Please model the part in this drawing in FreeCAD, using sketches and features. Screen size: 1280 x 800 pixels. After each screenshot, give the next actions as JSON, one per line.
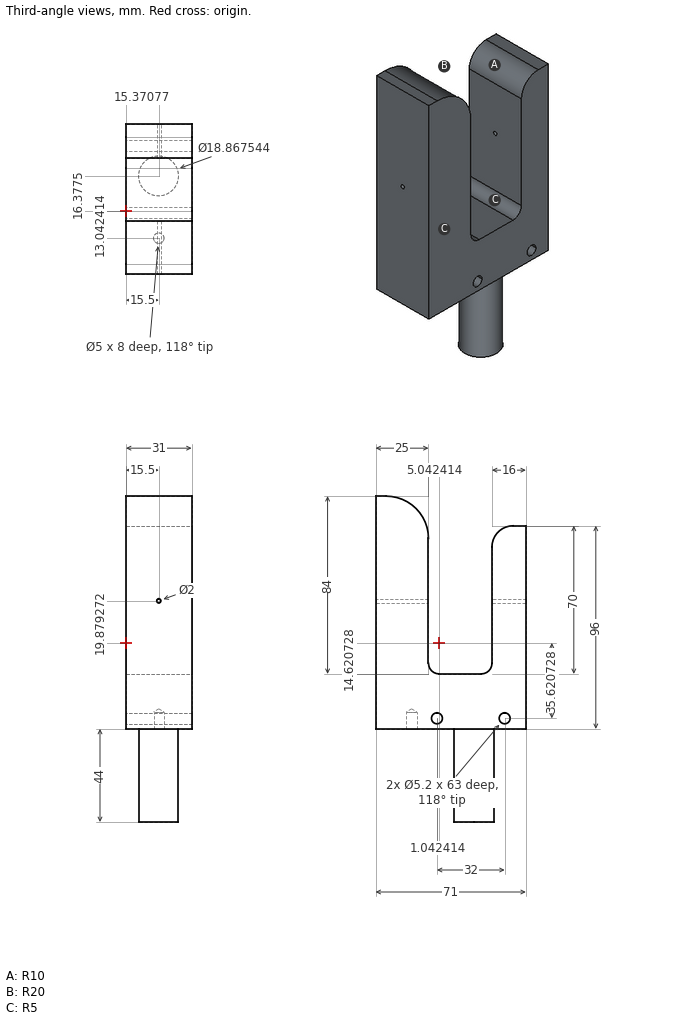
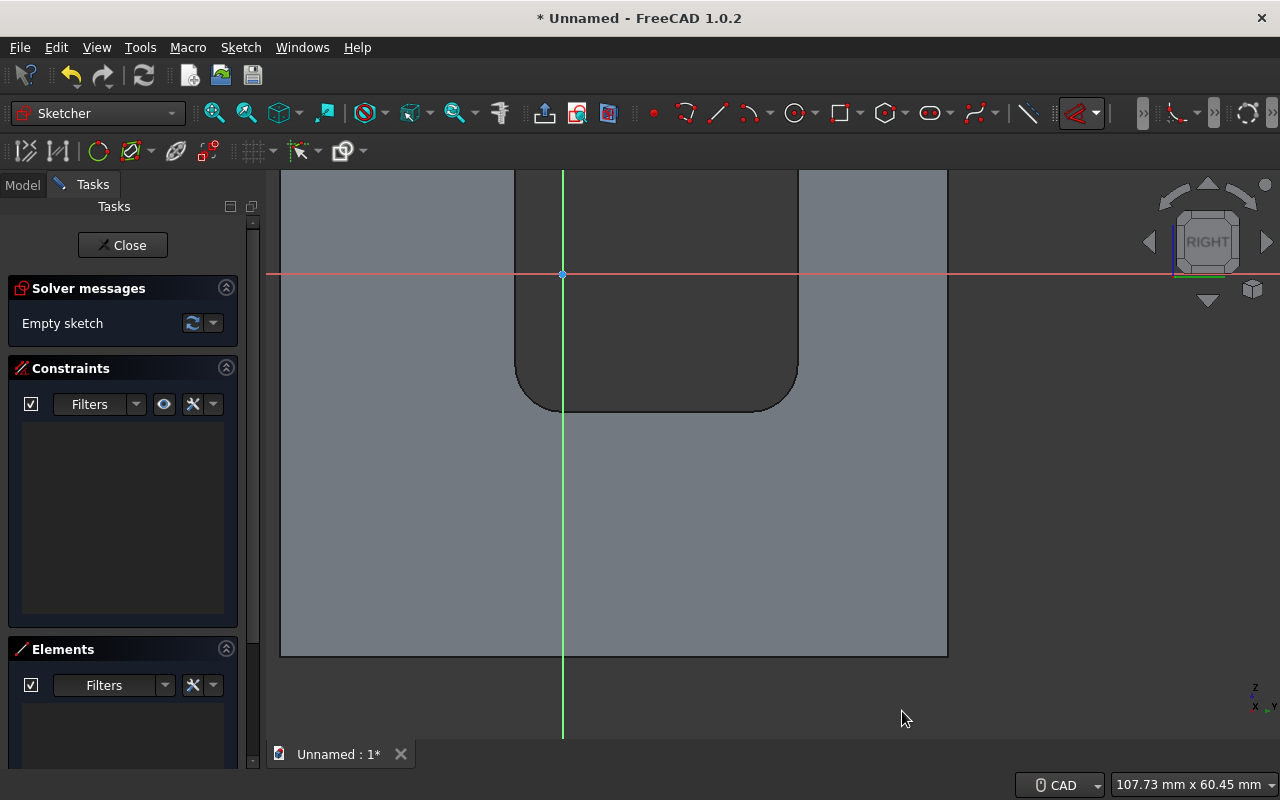
{"action": "left_click", "coordinate": [796, 114]}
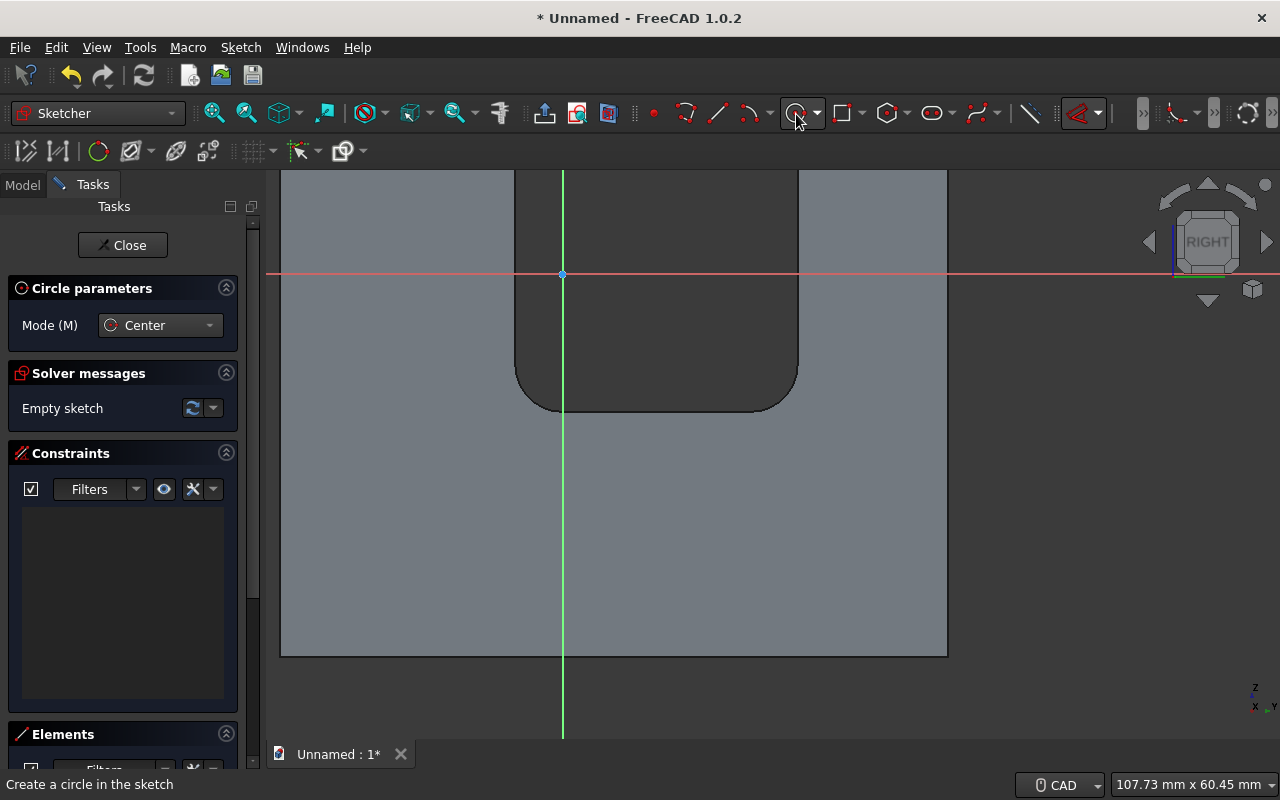
{"action": "left_click", "coordinate": [854, 610]}
{"action": "mouse_move", "coordinate": [871, 592]}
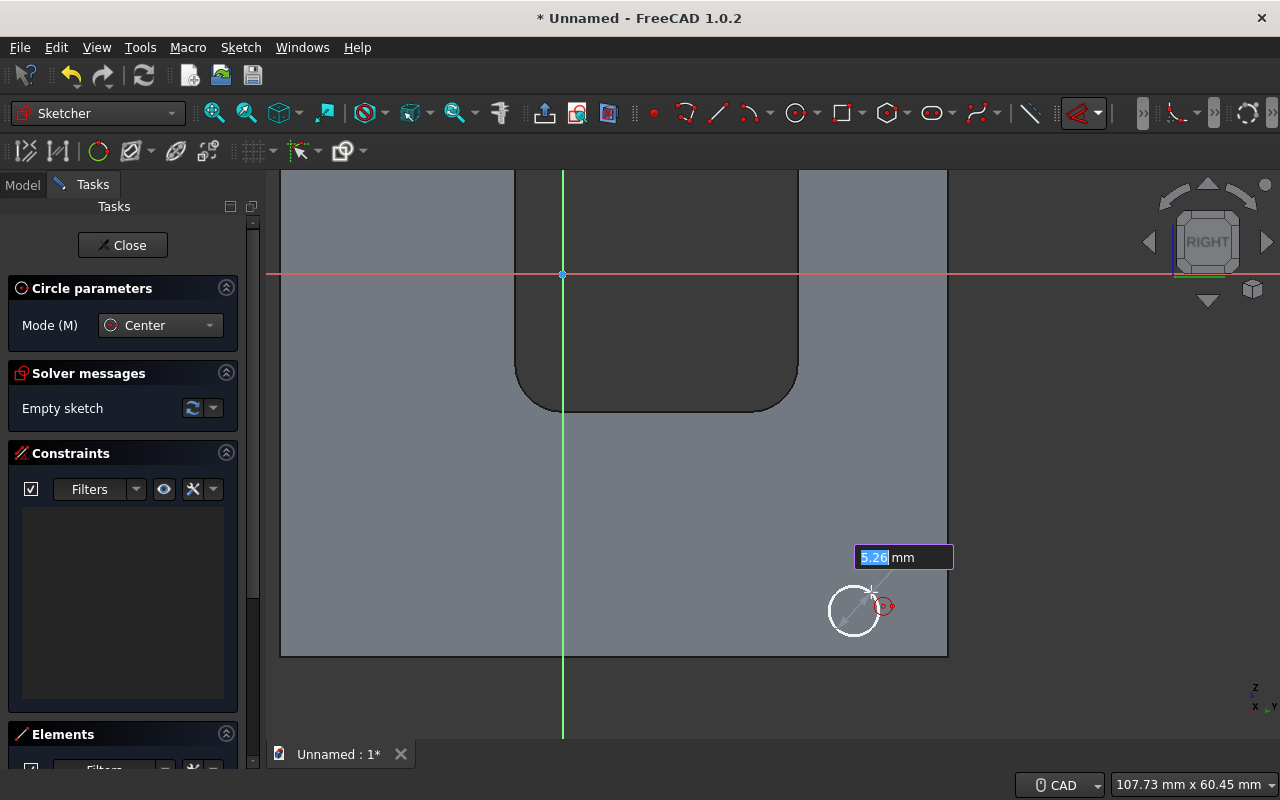
{"action": "type", "text": "5.2"}
{"action": "key", "text": "Return"}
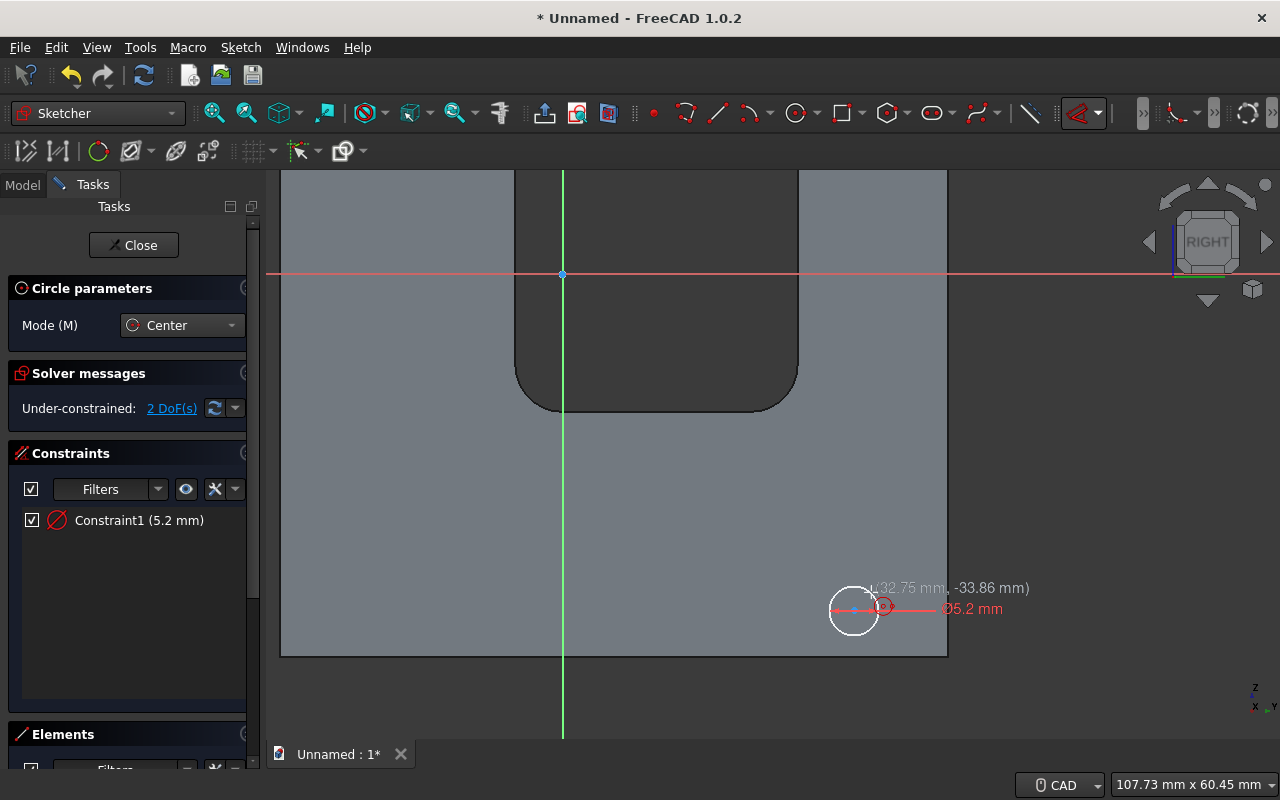
{"action": "scroll", "coordinate": [553, 610], "scroll_direction": "up", "scroll_amount": 3}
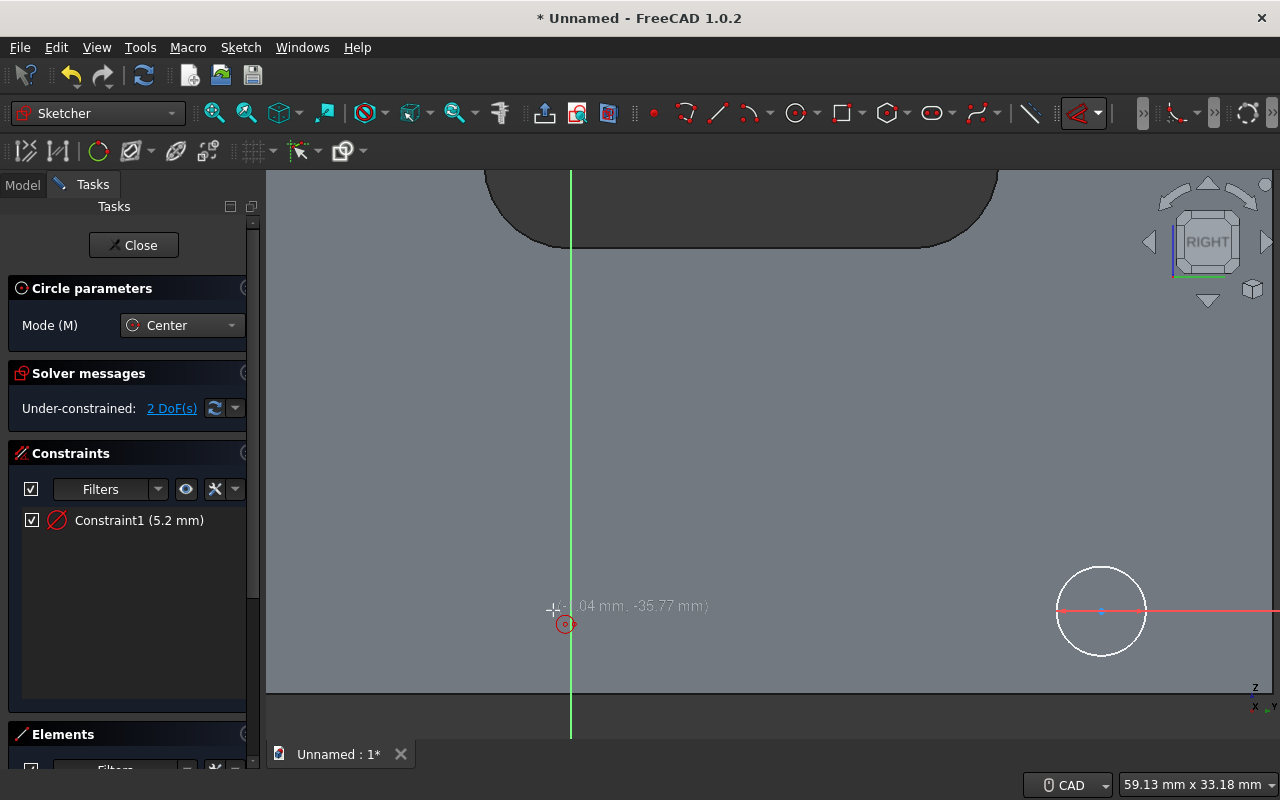
{"action": "left_click", "coordinate": [553, 609]}
{"action": "mouse_move", "coordinate": [521, 577]}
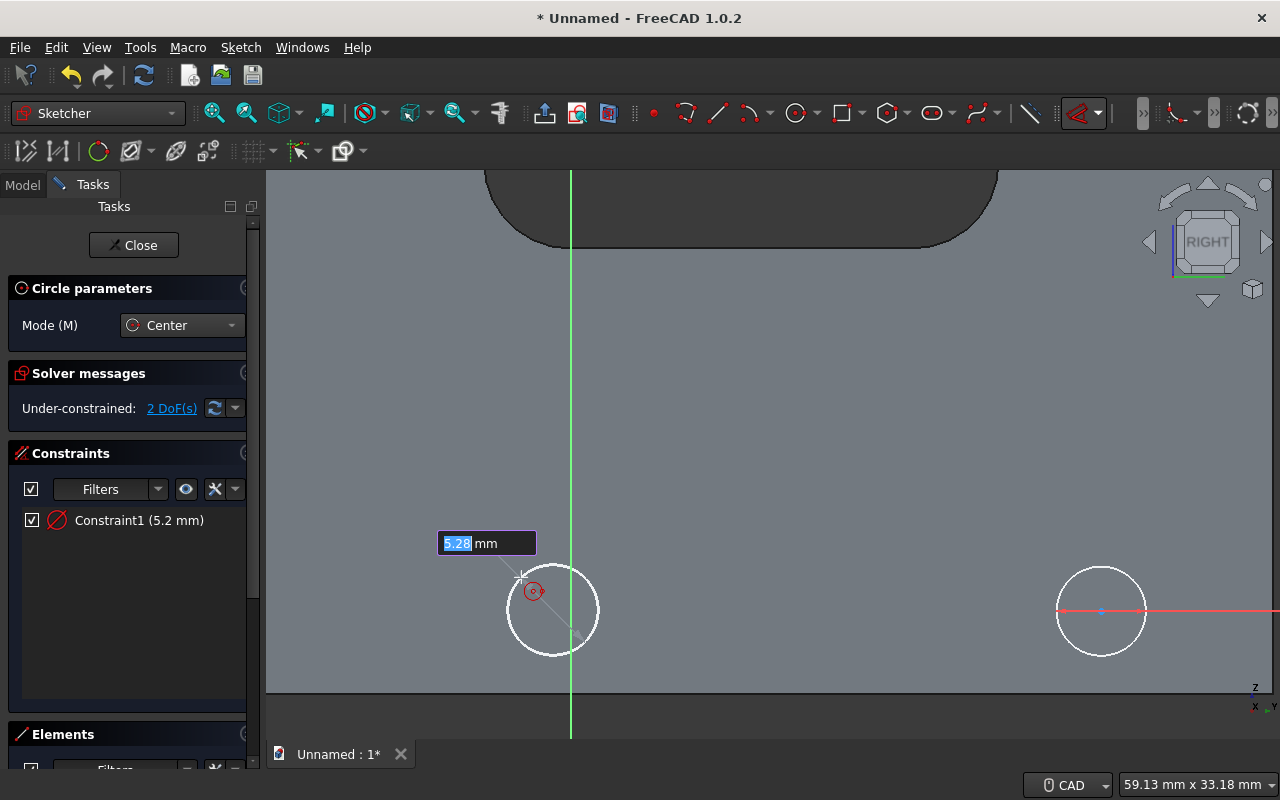
{"action": "type", "text": "5.2"}
{"action": "key", "text": "Return"}
{"action": "key", "text": "Escape"}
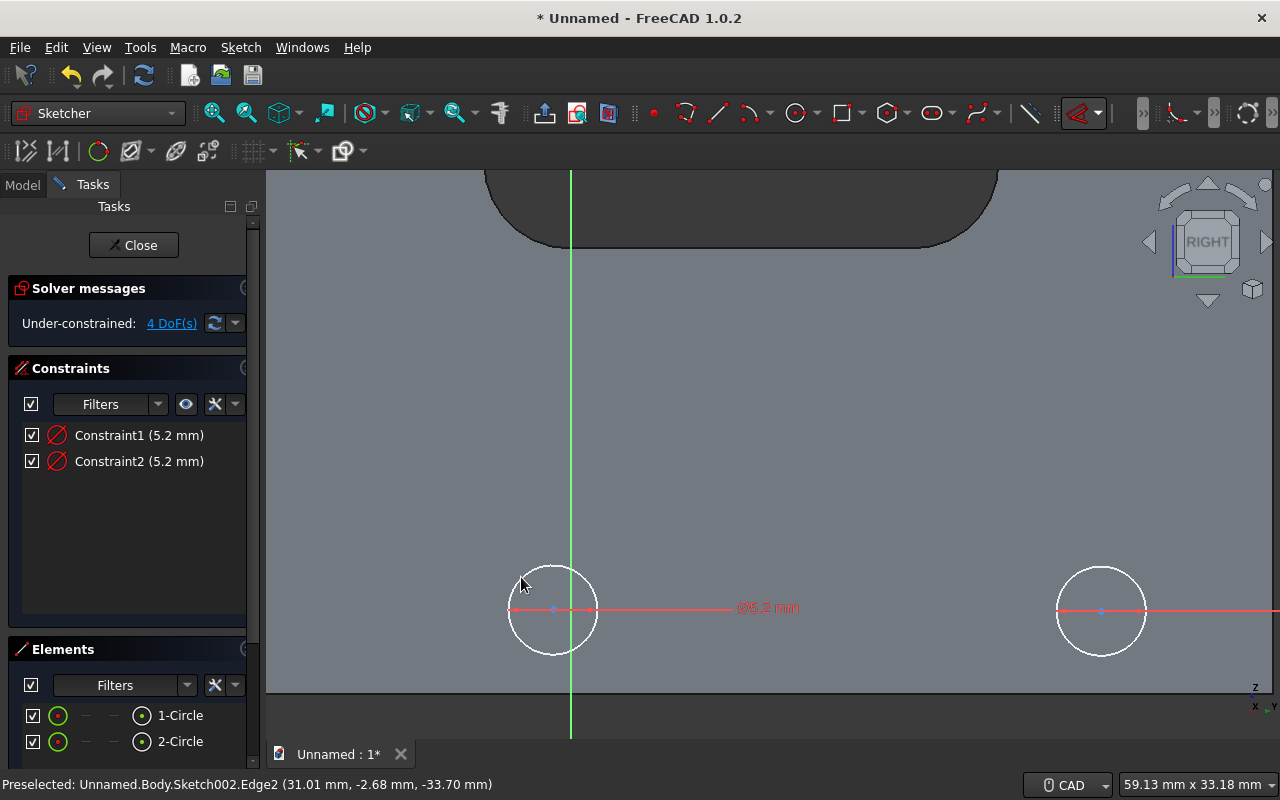
{"action": "left_click", "coordinate": [1101, 611]}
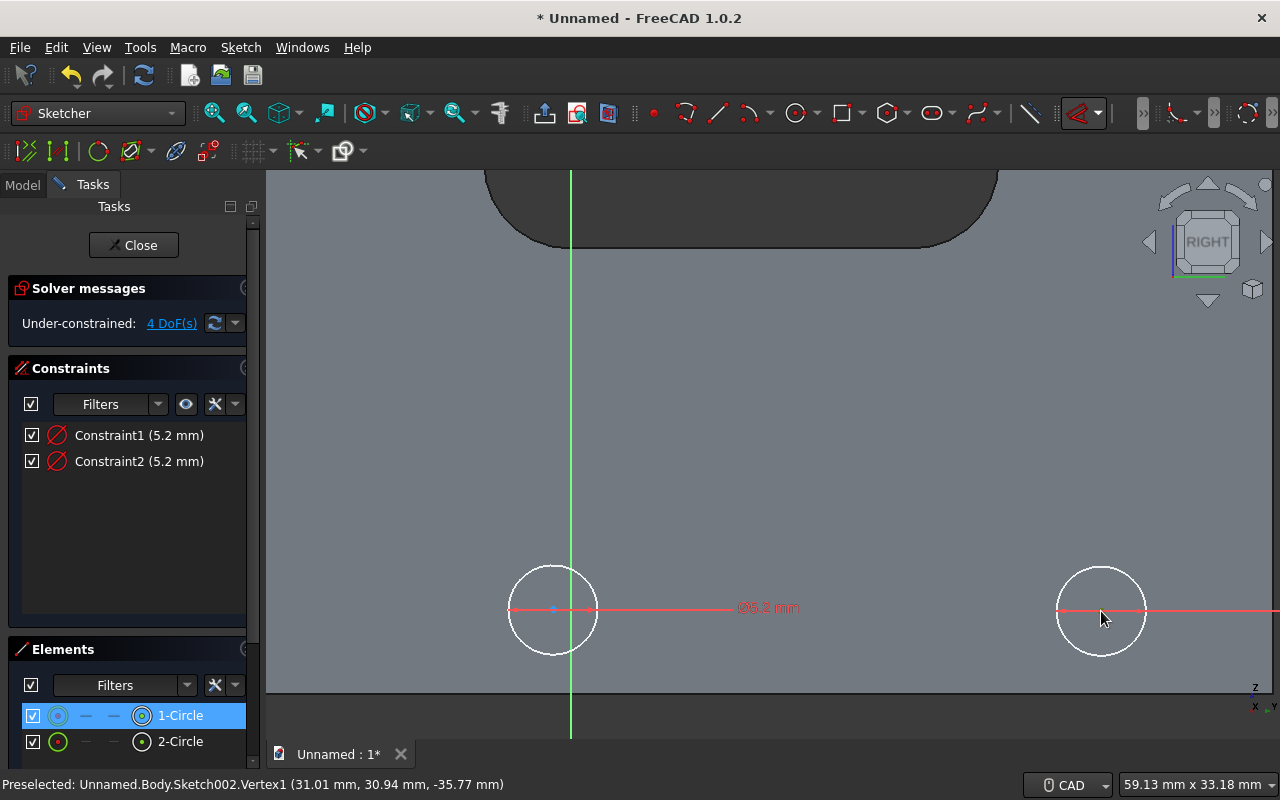
{"action": "left_click", "coordinate": [553, 610]}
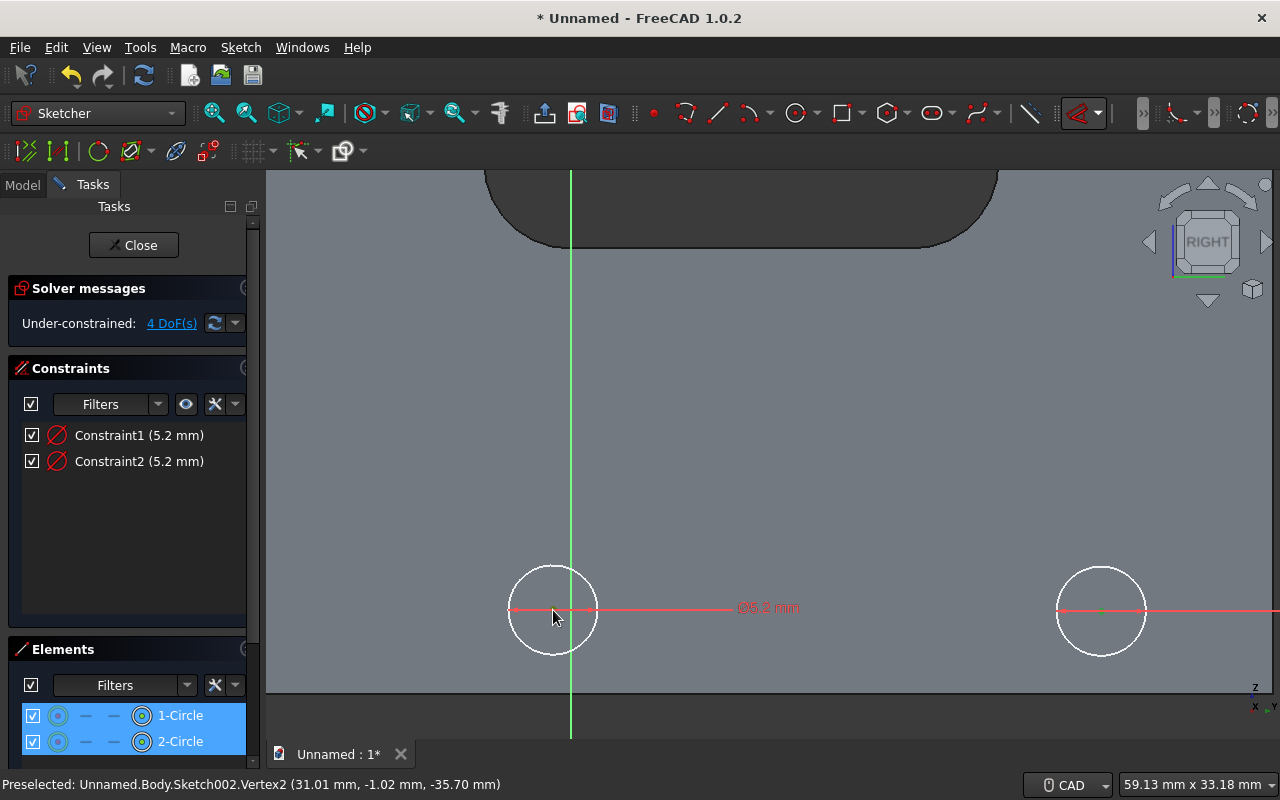
{"action": "key", "text": "h"}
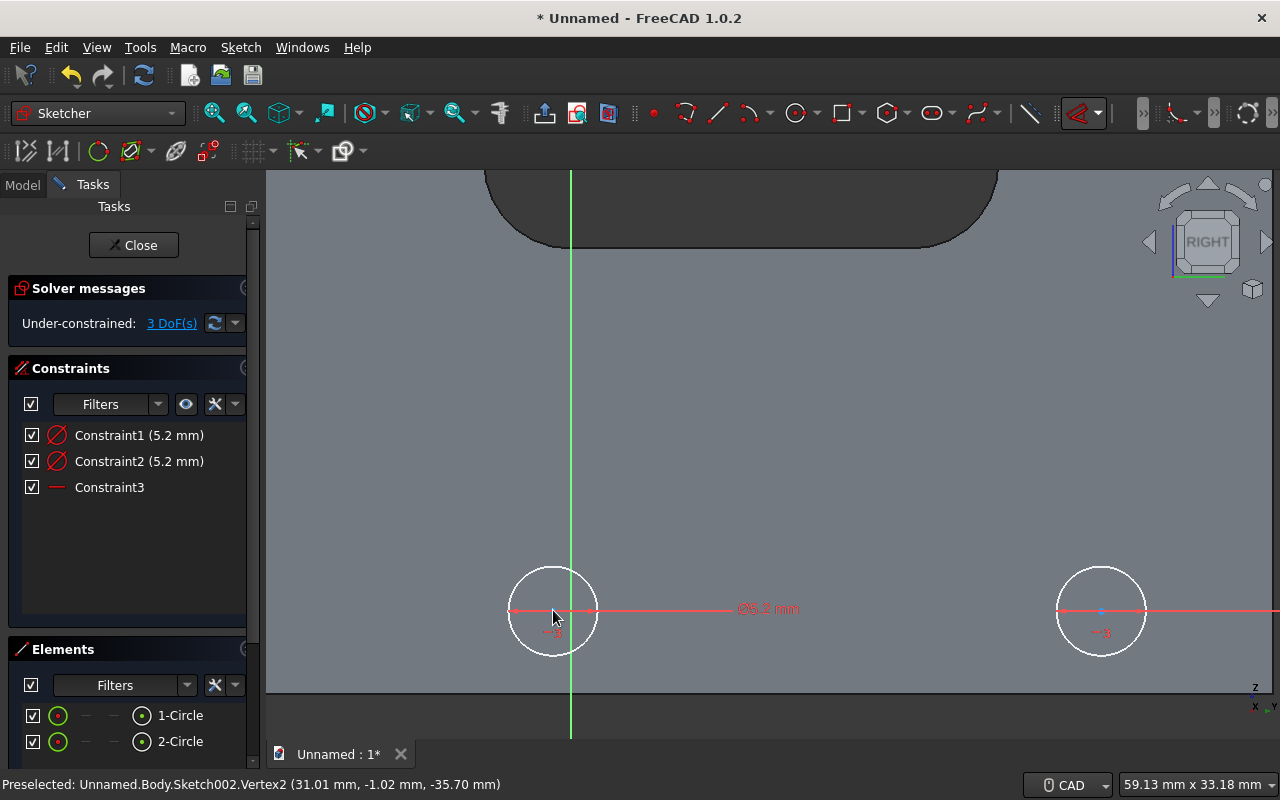
{"action": "left_click", "coordinate": [1101, 611]}